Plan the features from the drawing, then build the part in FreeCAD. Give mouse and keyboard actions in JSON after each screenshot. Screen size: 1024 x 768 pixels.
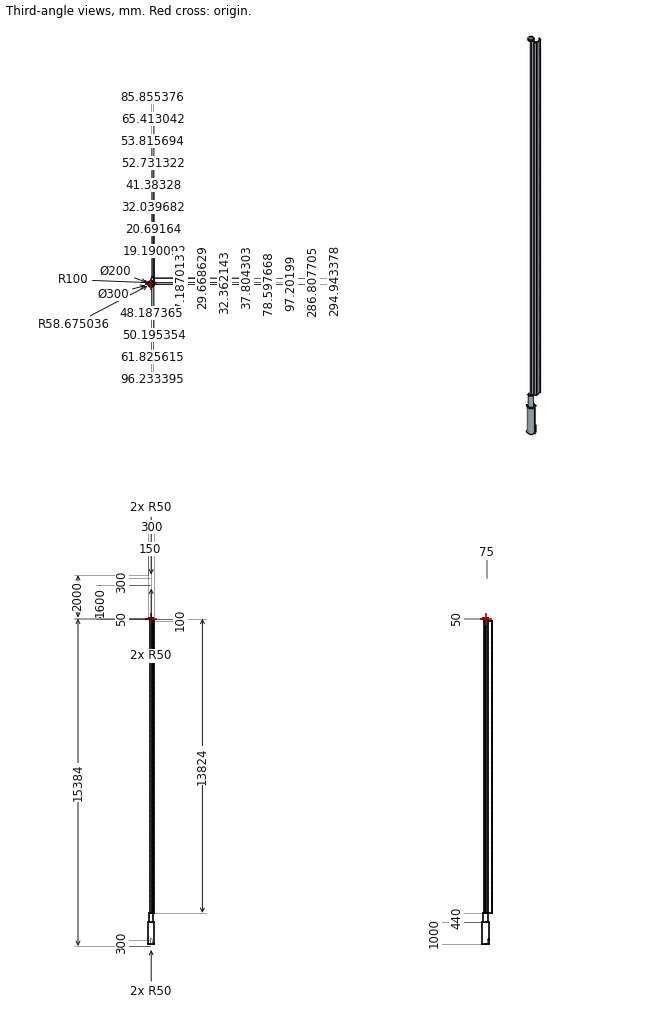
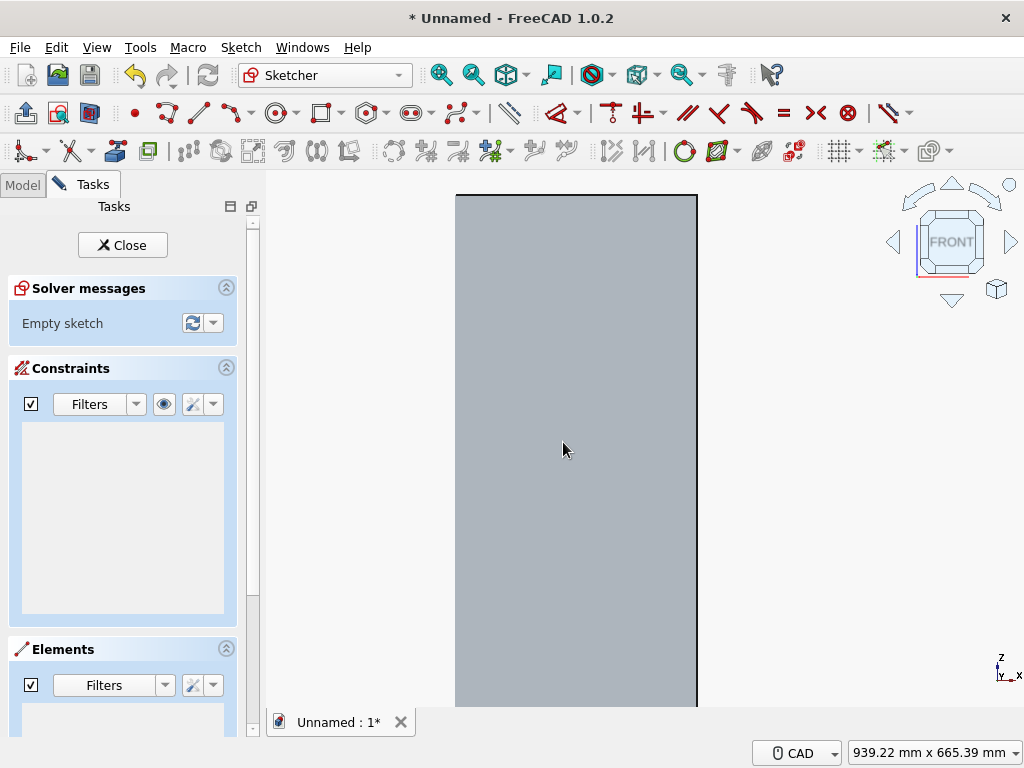
{"action": "left_click", "coordinate": [412, 114]}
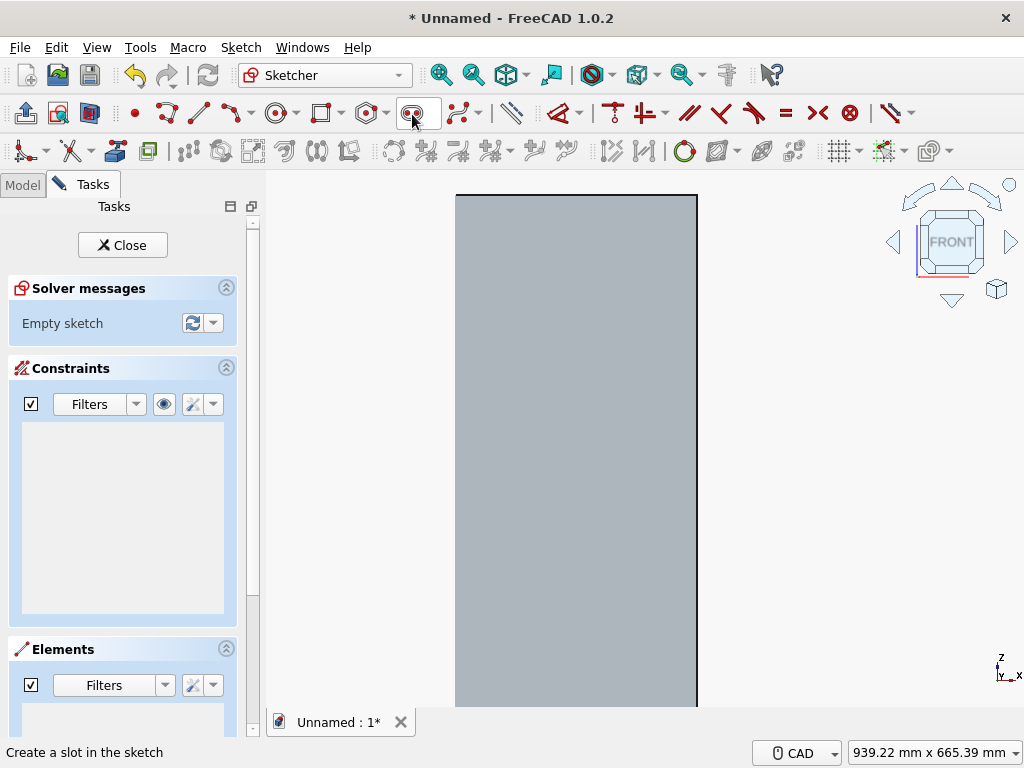
{"action": "left_click", "coordinate": [576, 558]}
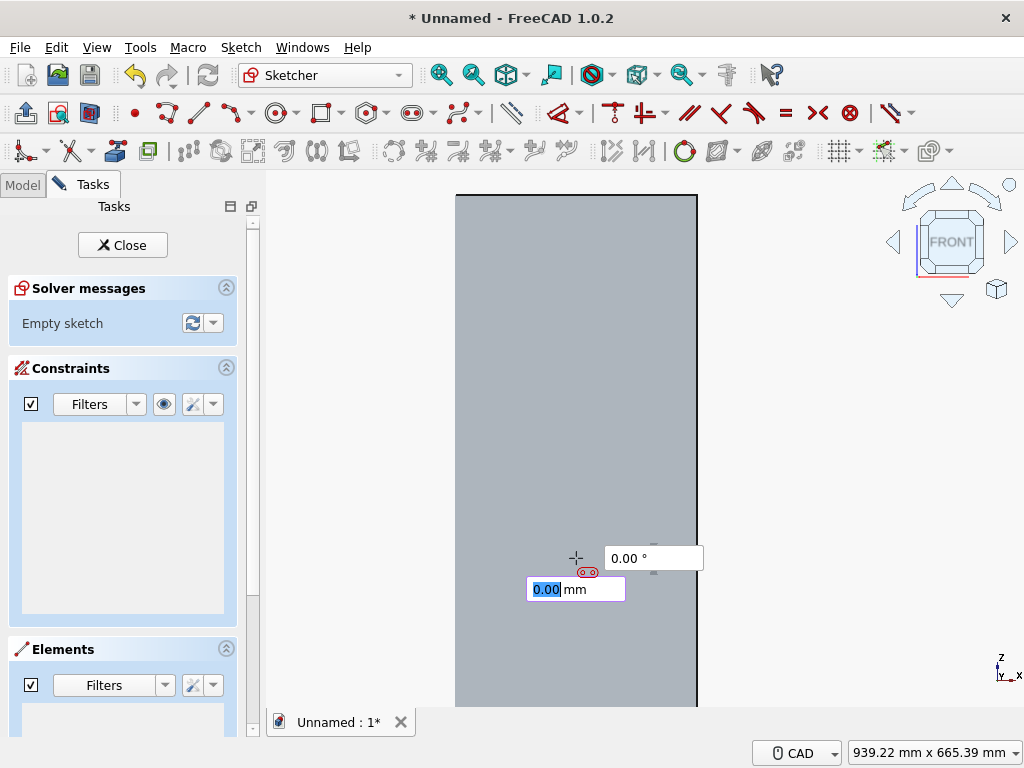
{"action": "left_click", "coordinate": [585, 316]}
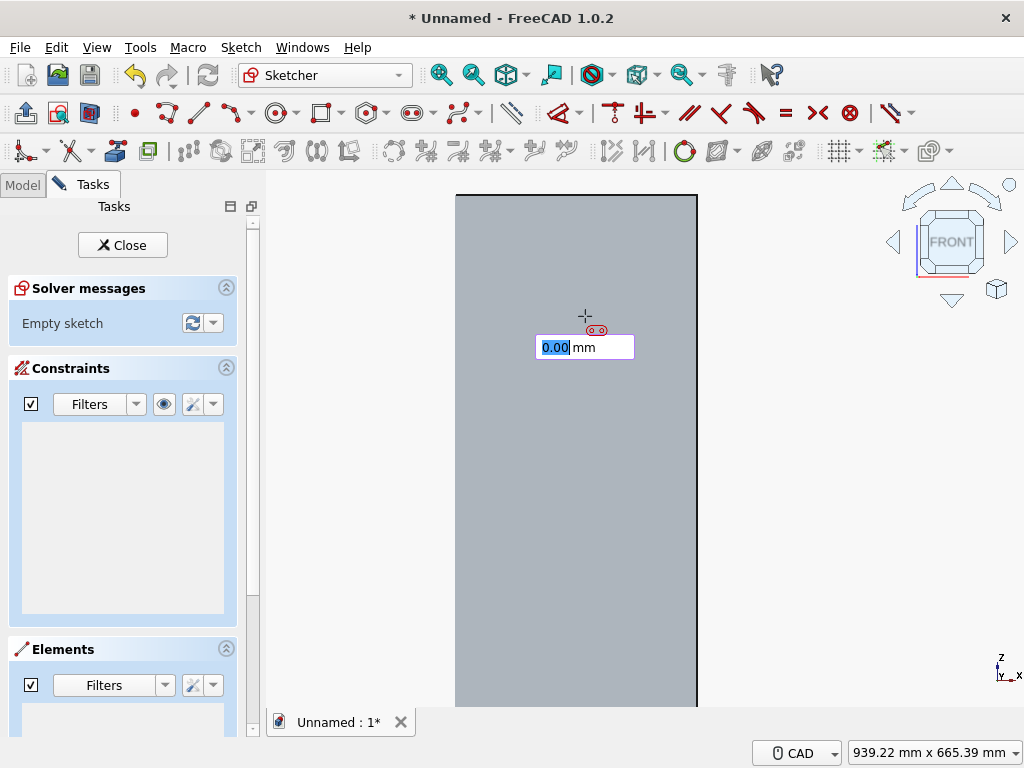
{"action": "left_click", "coordinate": [617, 437]}
{"action": "key", "text": "Escape"}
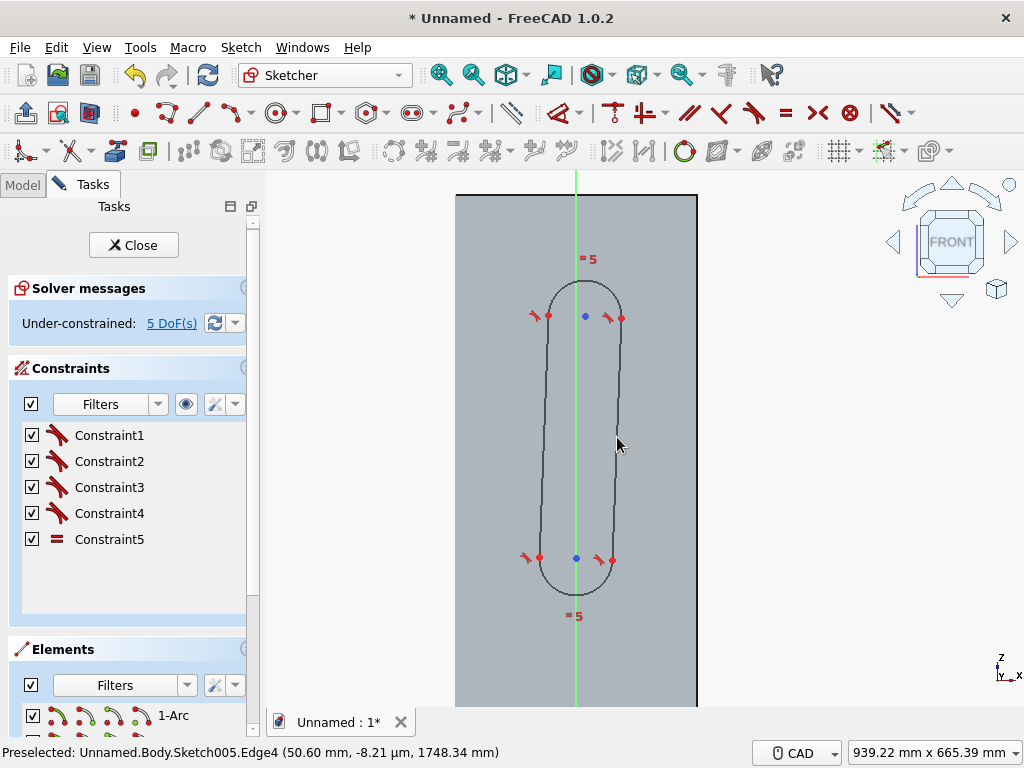
{"action": "left_click", "coordinate": [542, 485]}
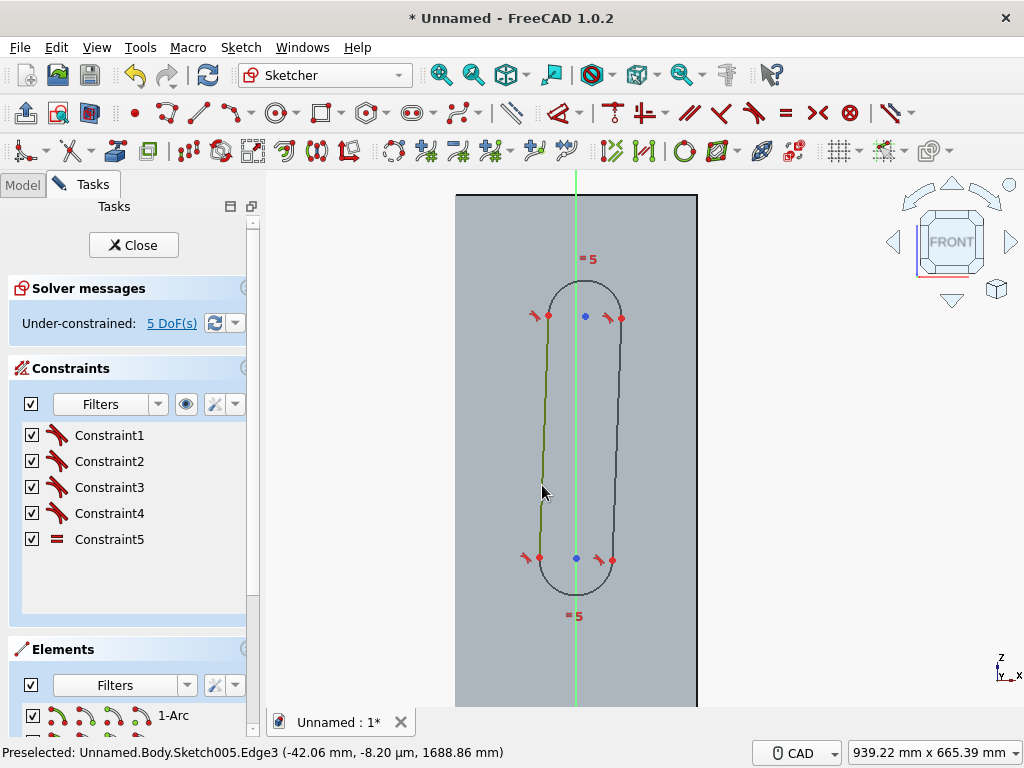
{"action": "key", "text": "v"}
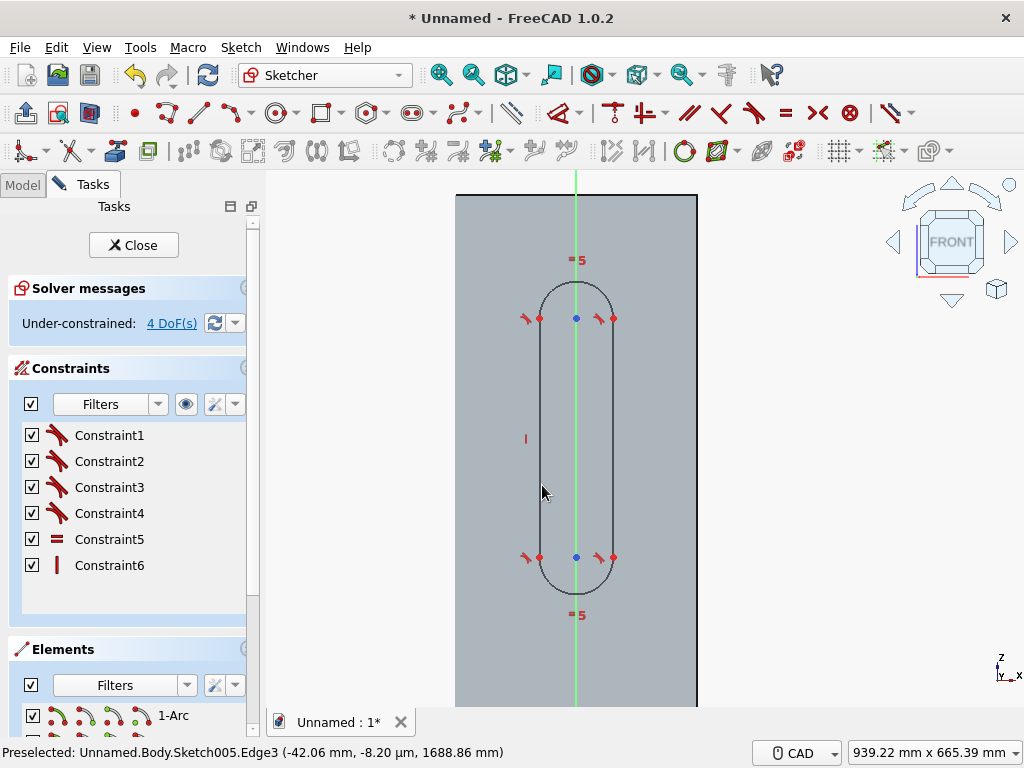
{"action": "left_click", "coordinate": [576, 558]}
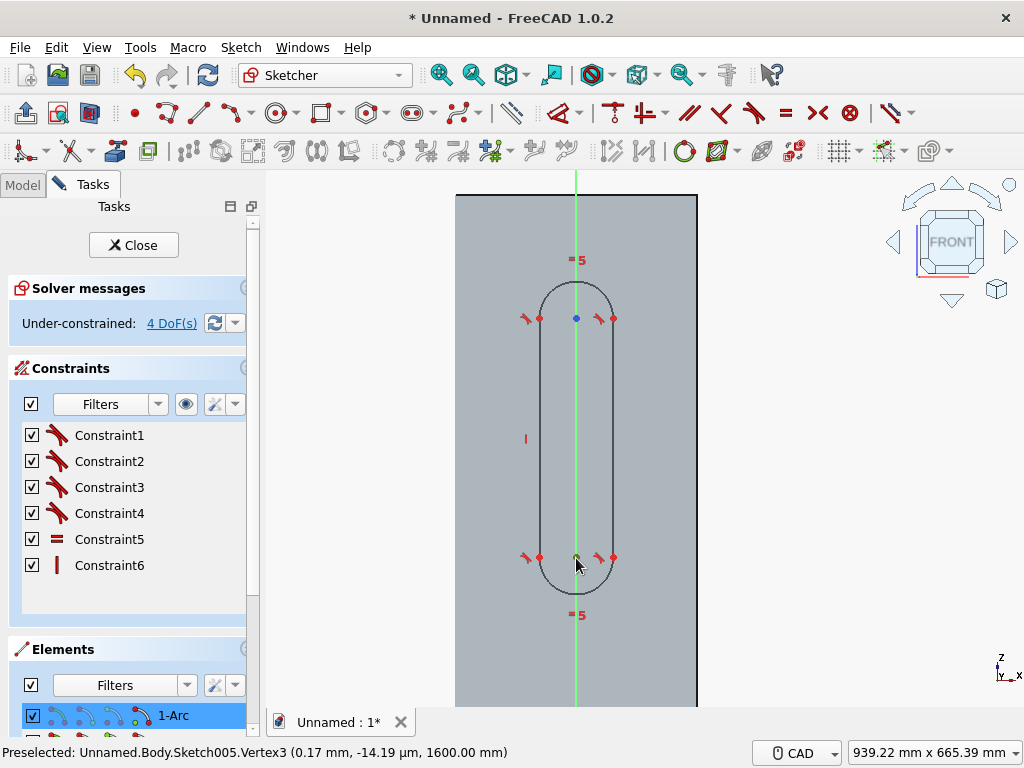
{"action": "left_click", "coordinate": [576, 645]}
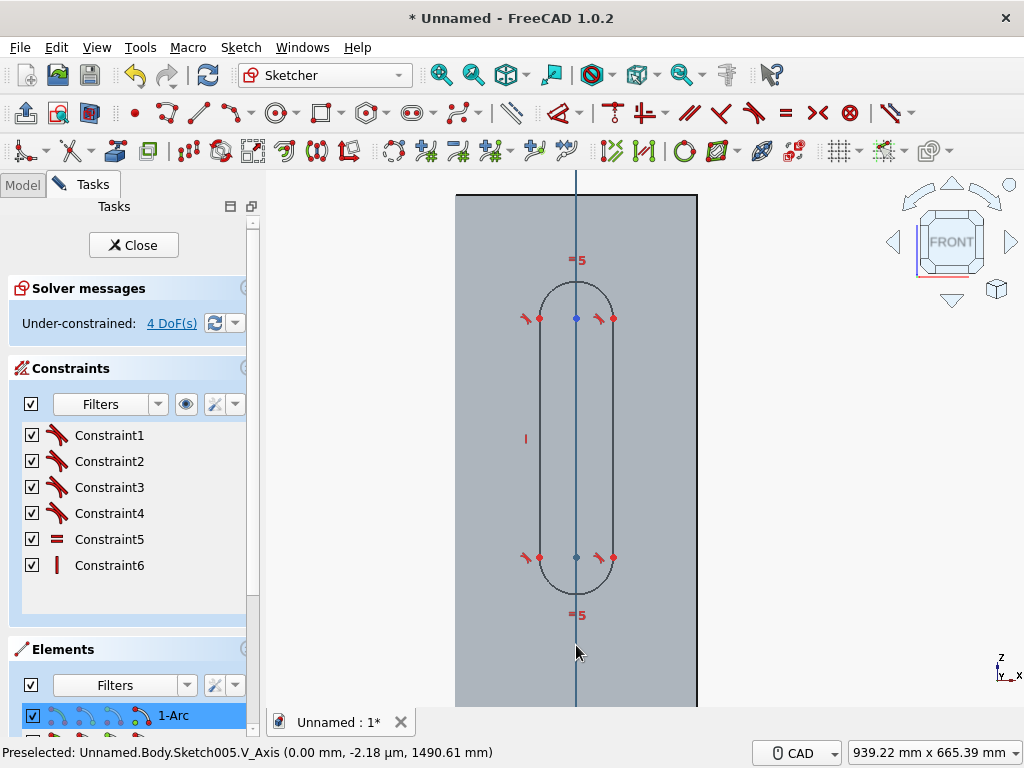
{"action": "left_click", "coordinate": [614, 114]}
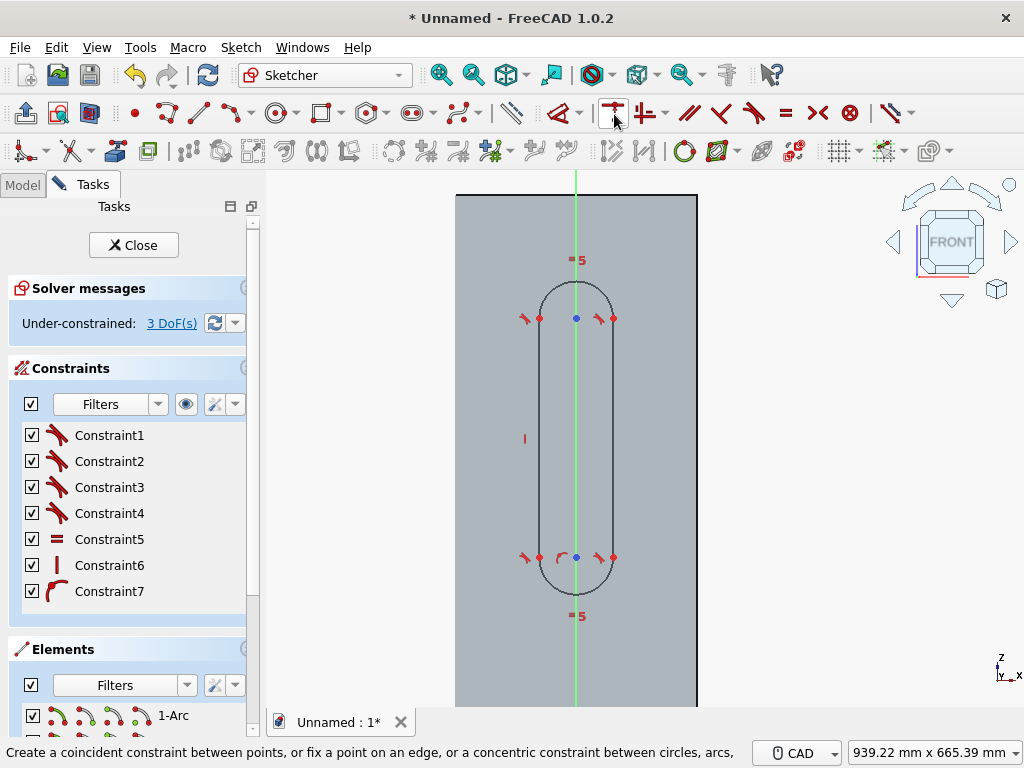
{"action": "left_click", "coordinate": [558, 114]}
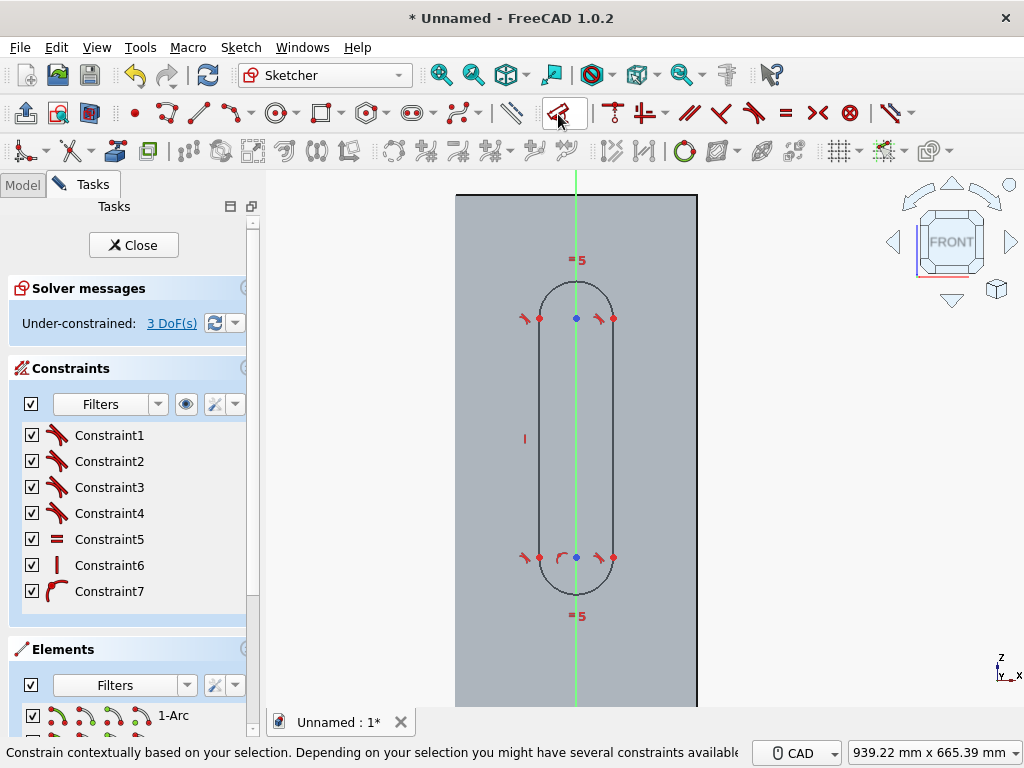
{"action": "left_click", "coordinate": [554, 588]}
{"action": "left_click", "coordinate": [535, 614]}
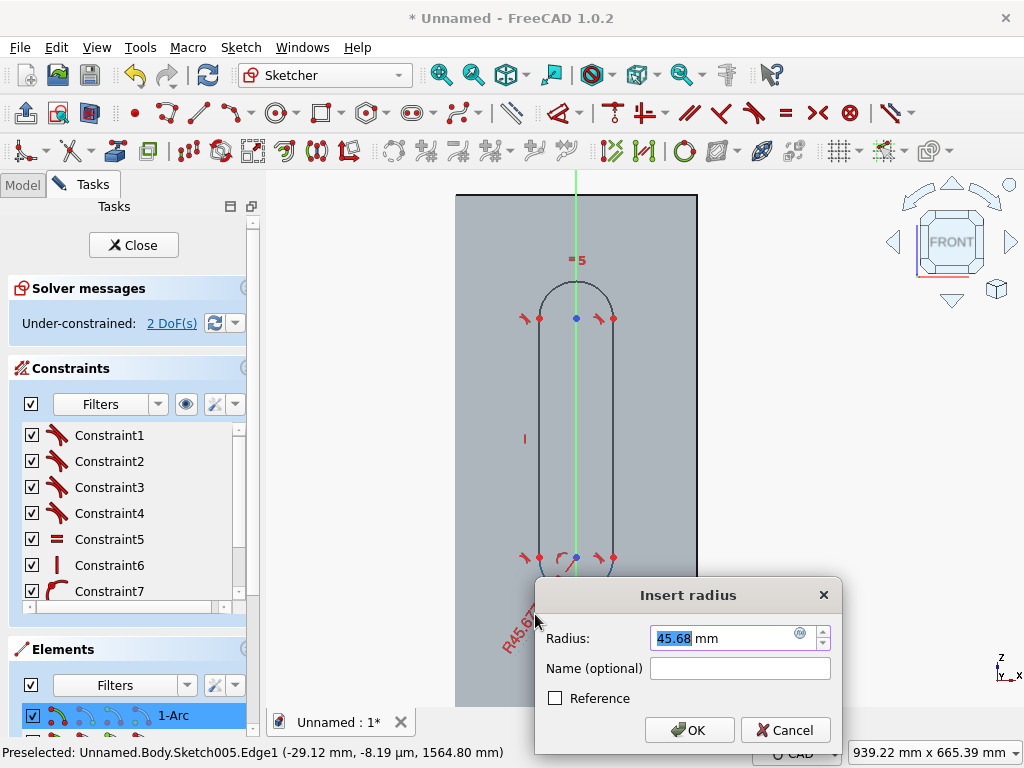
{"action": "type", "text": "50"}
{"action": "key", "text": "Return"}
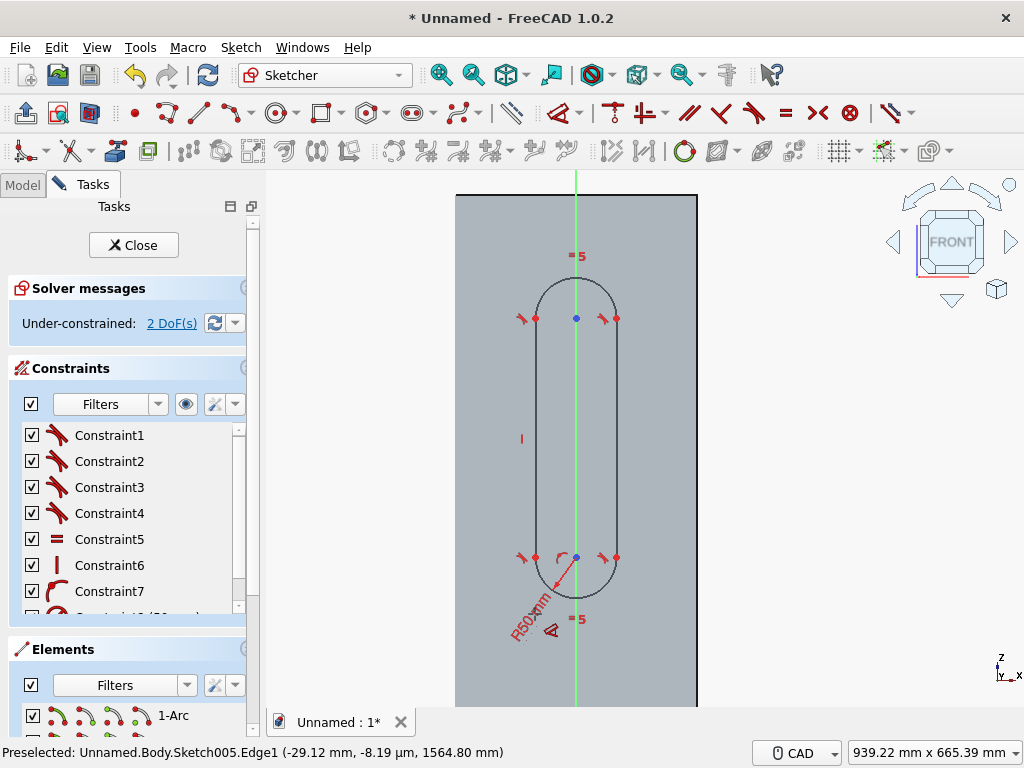
{"action": "left_click", "coordinate": [536, 486]}
{"action": "left_click", "coordinate": [502, 438]}